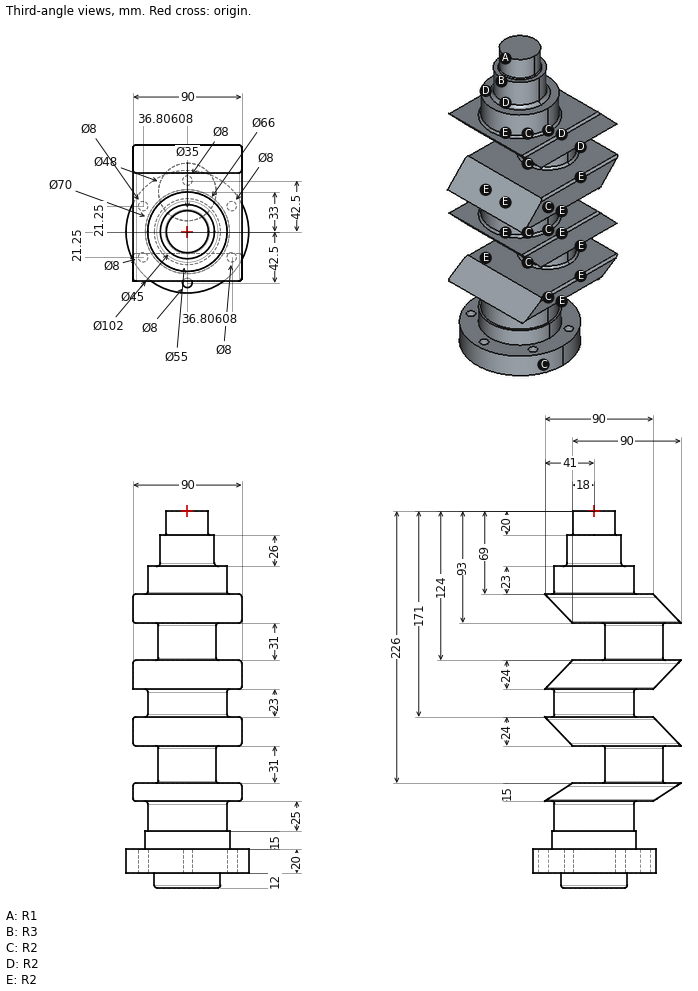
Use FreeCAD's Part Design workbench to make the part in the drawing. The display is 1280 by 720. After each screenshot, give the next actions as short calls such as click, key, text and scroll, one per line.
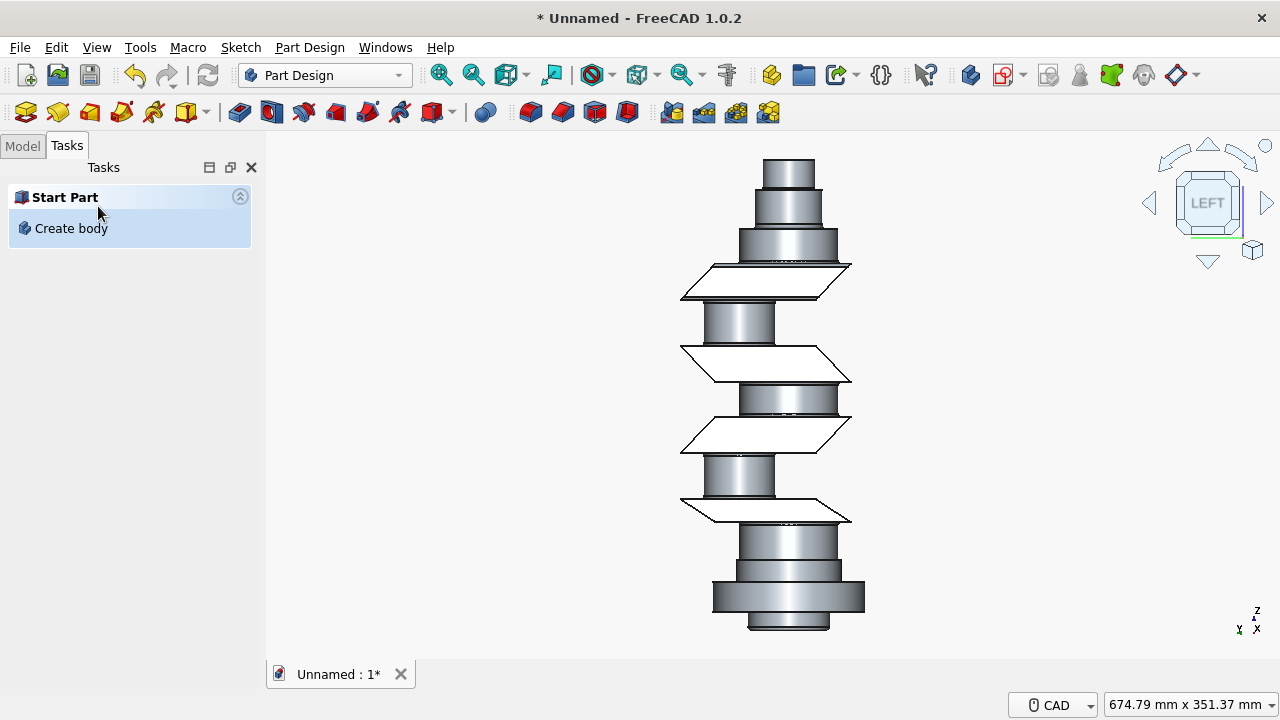
click(748, 345)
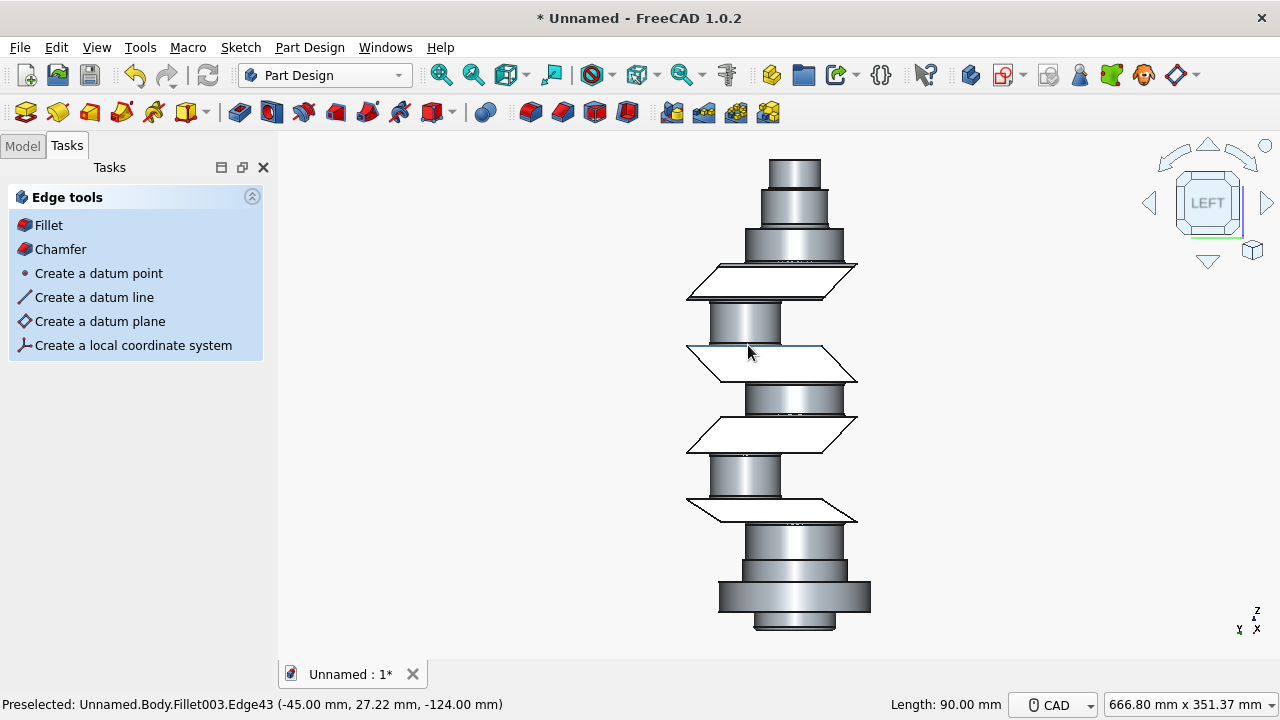
click(754, 452, ctrl)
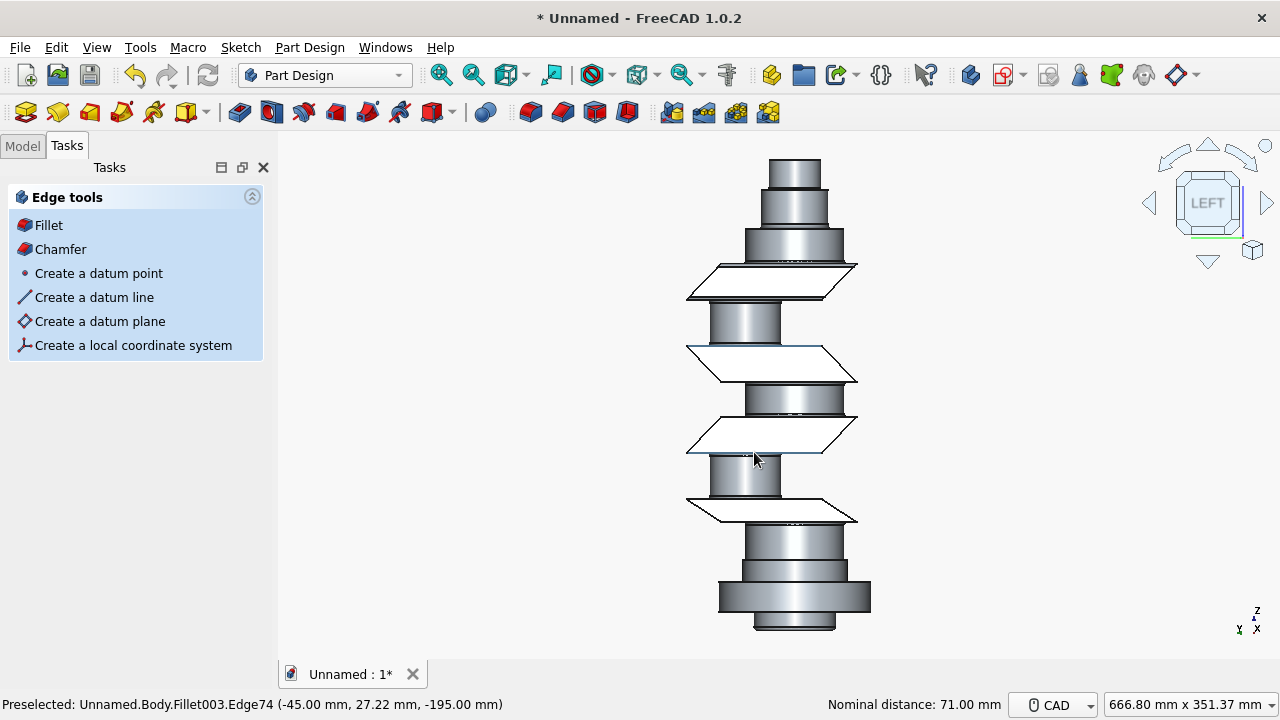
click(789, 416, ctrl)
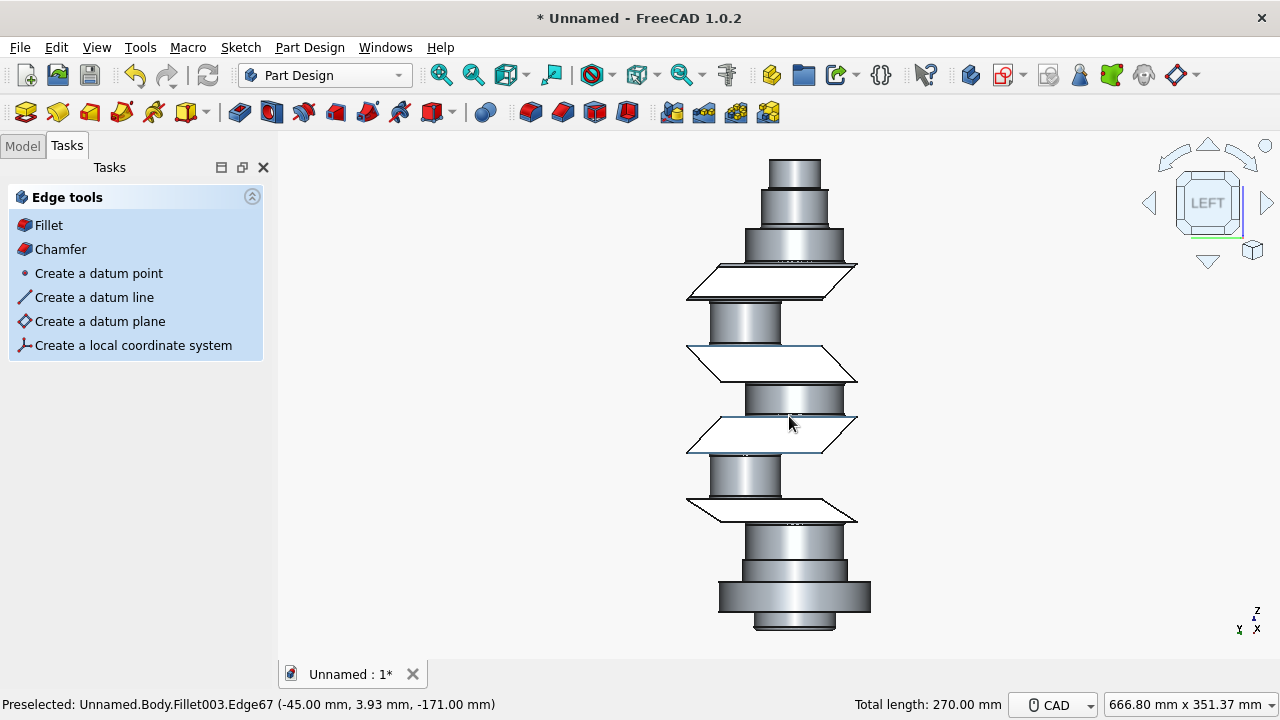
click(789, 521, ctrl)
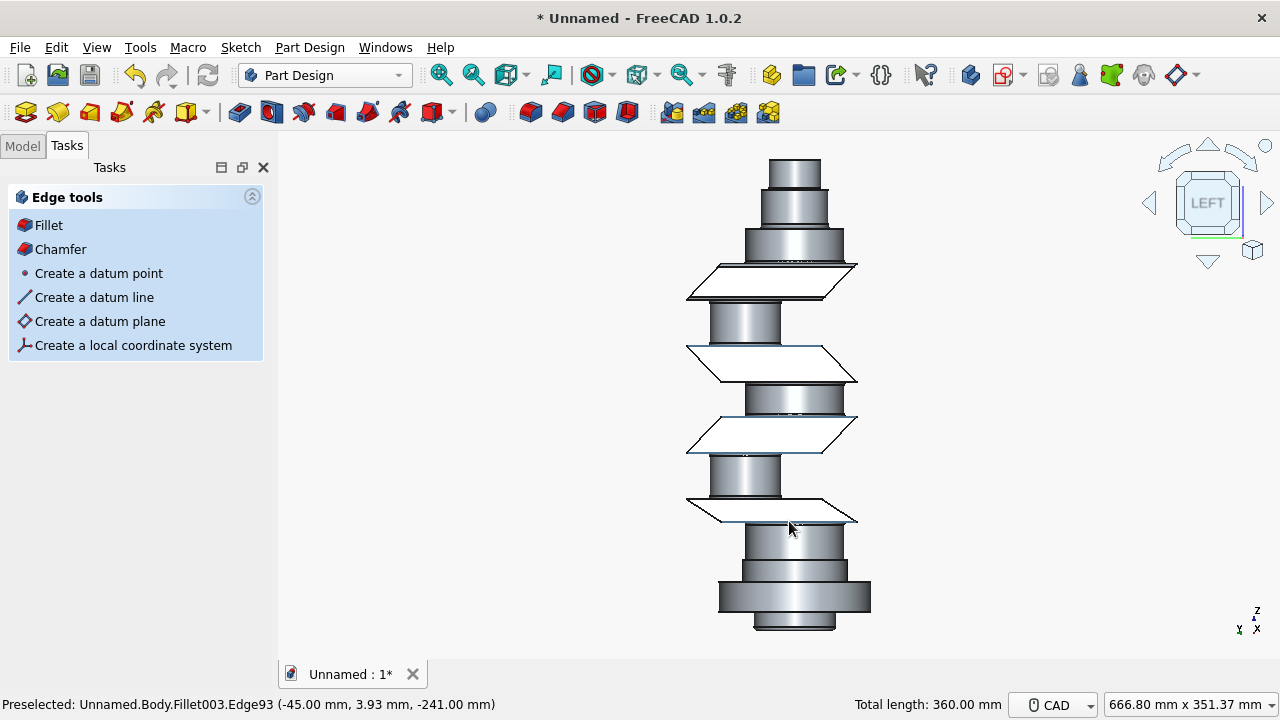
click(754, 498, ctrl)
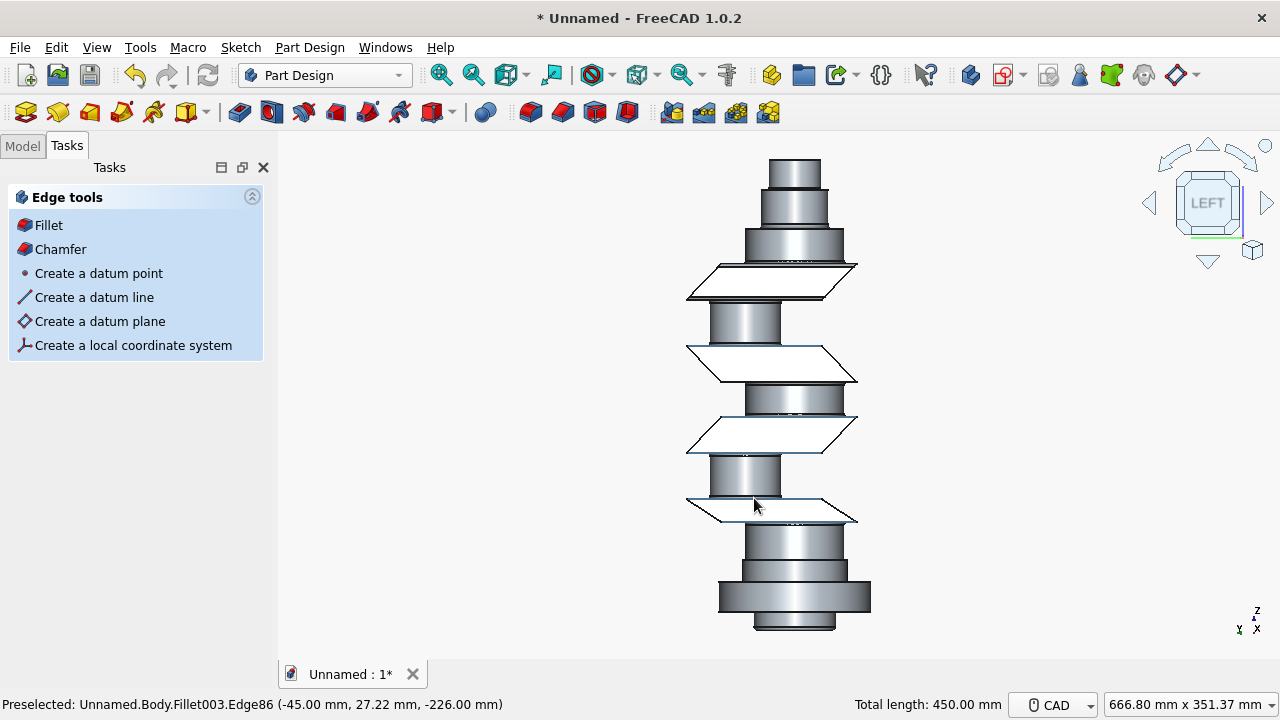
key(0)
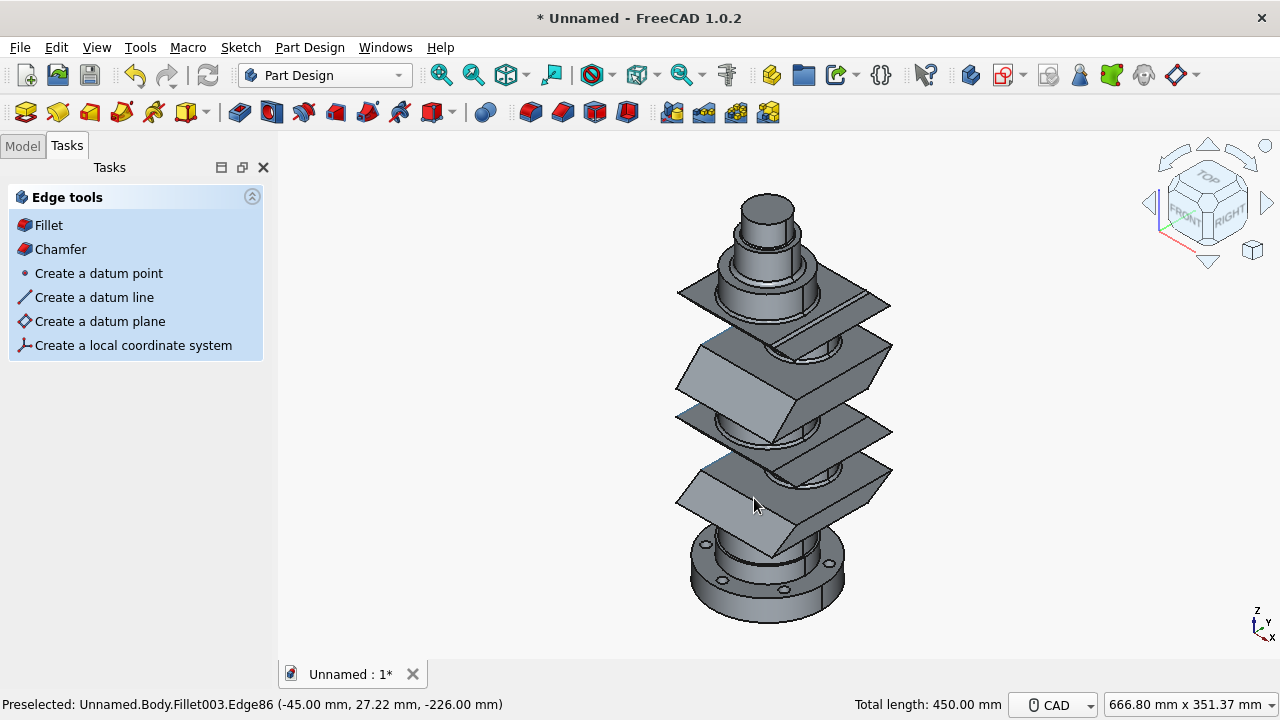
click(844, 372, ctrl)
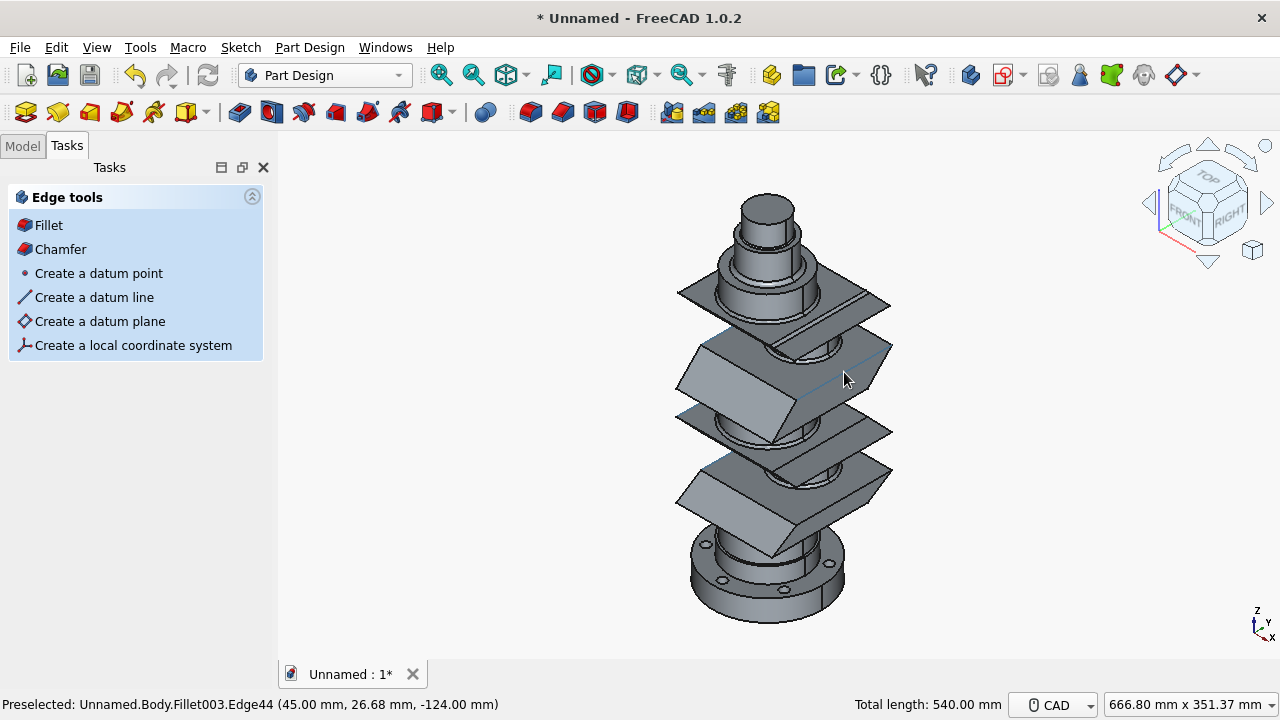
click(820, 443, ctrl)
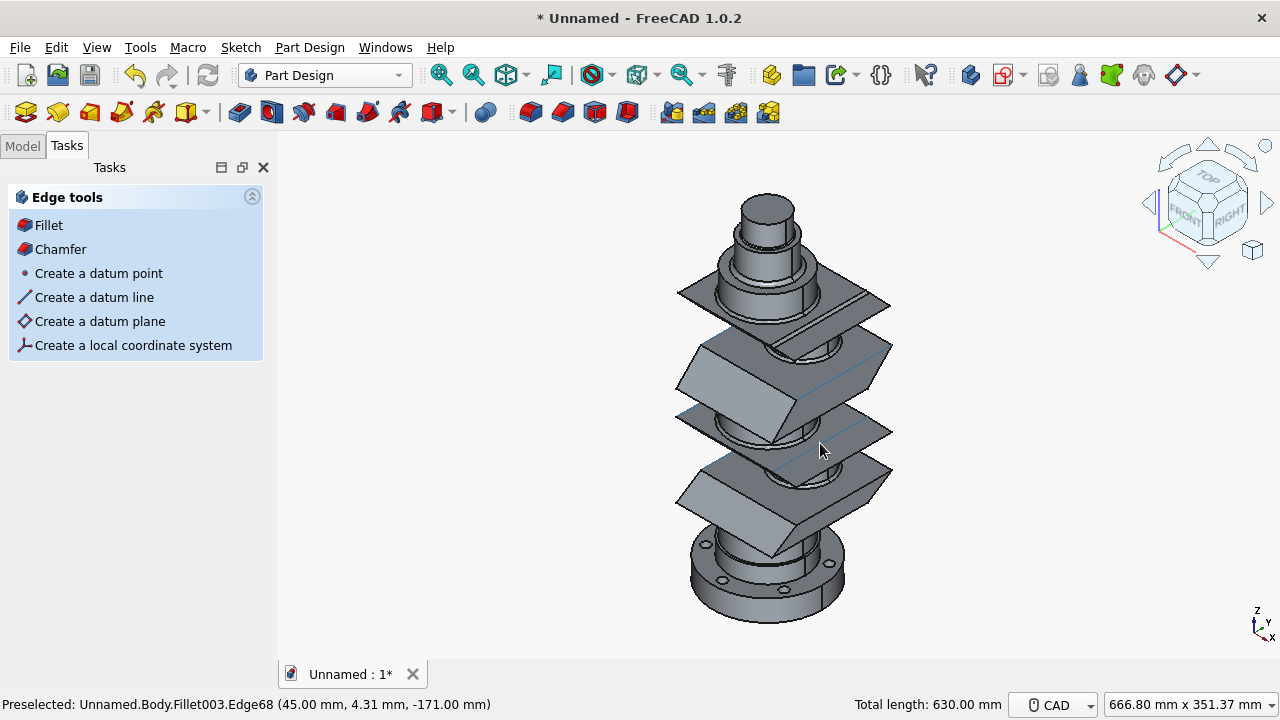
click(844, 497, ctrl)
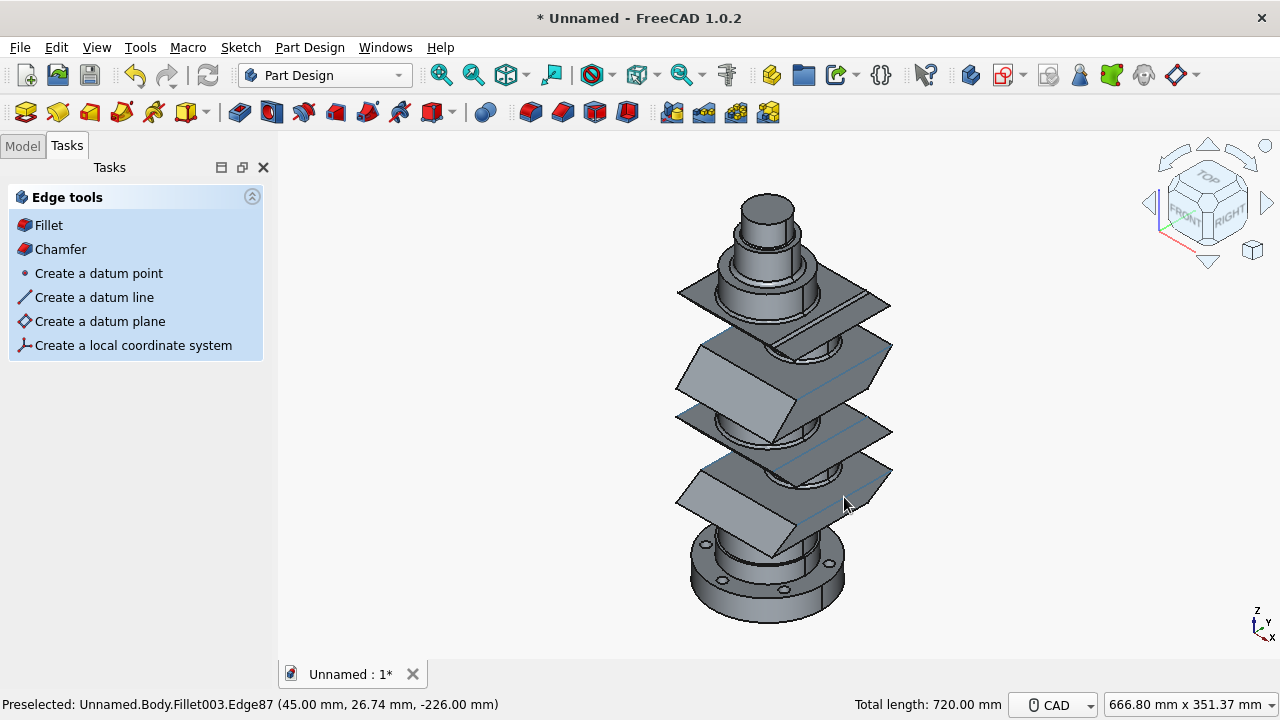
key(2)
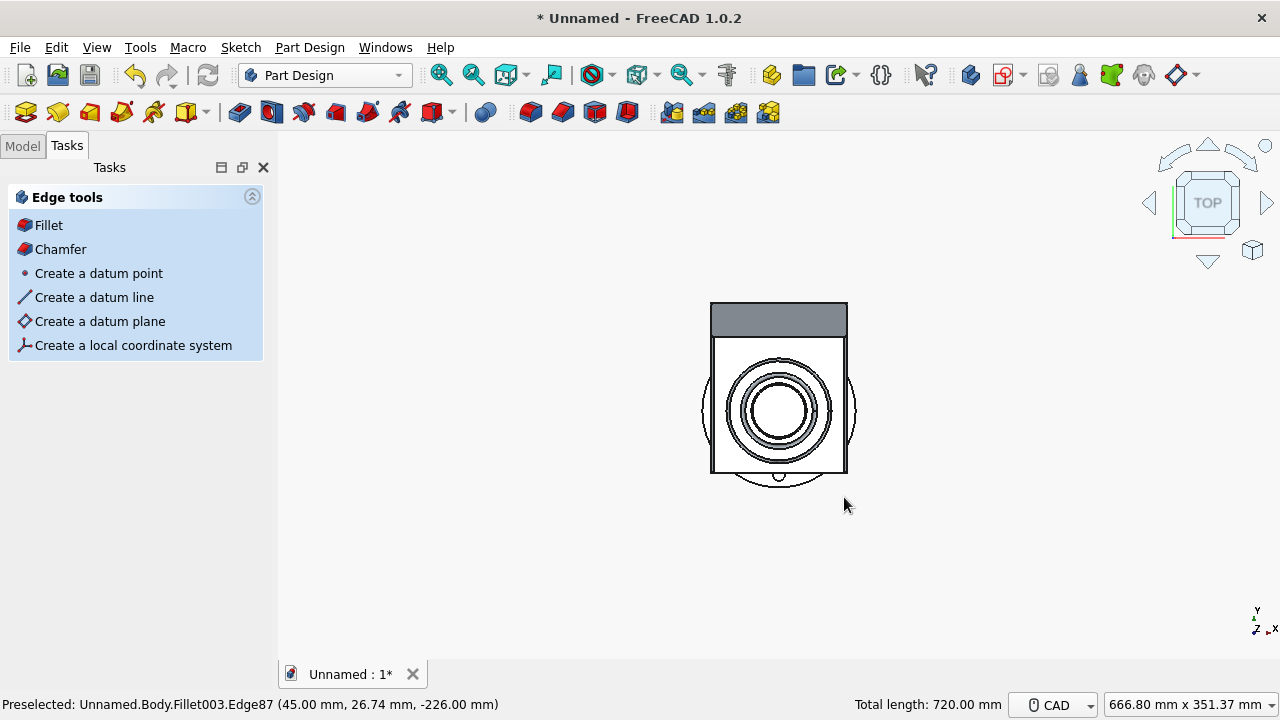
click(442, 76)